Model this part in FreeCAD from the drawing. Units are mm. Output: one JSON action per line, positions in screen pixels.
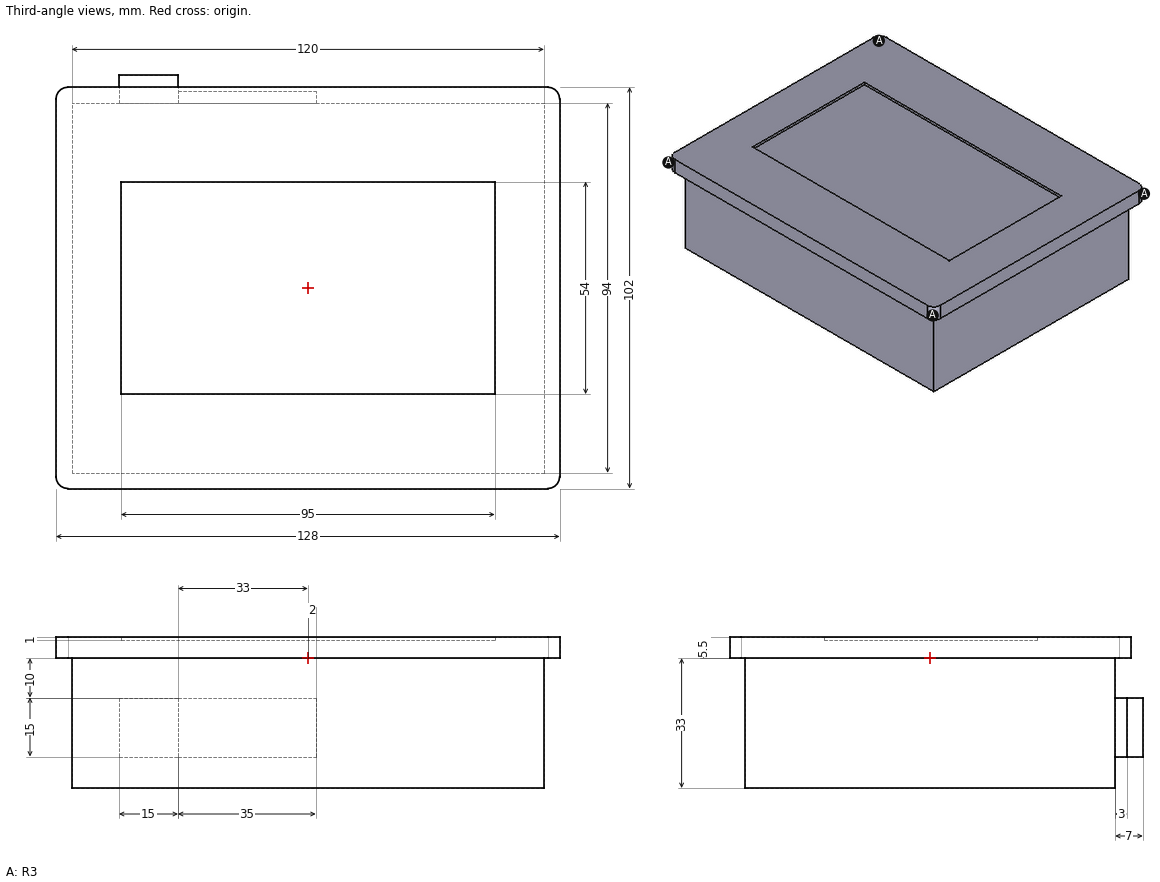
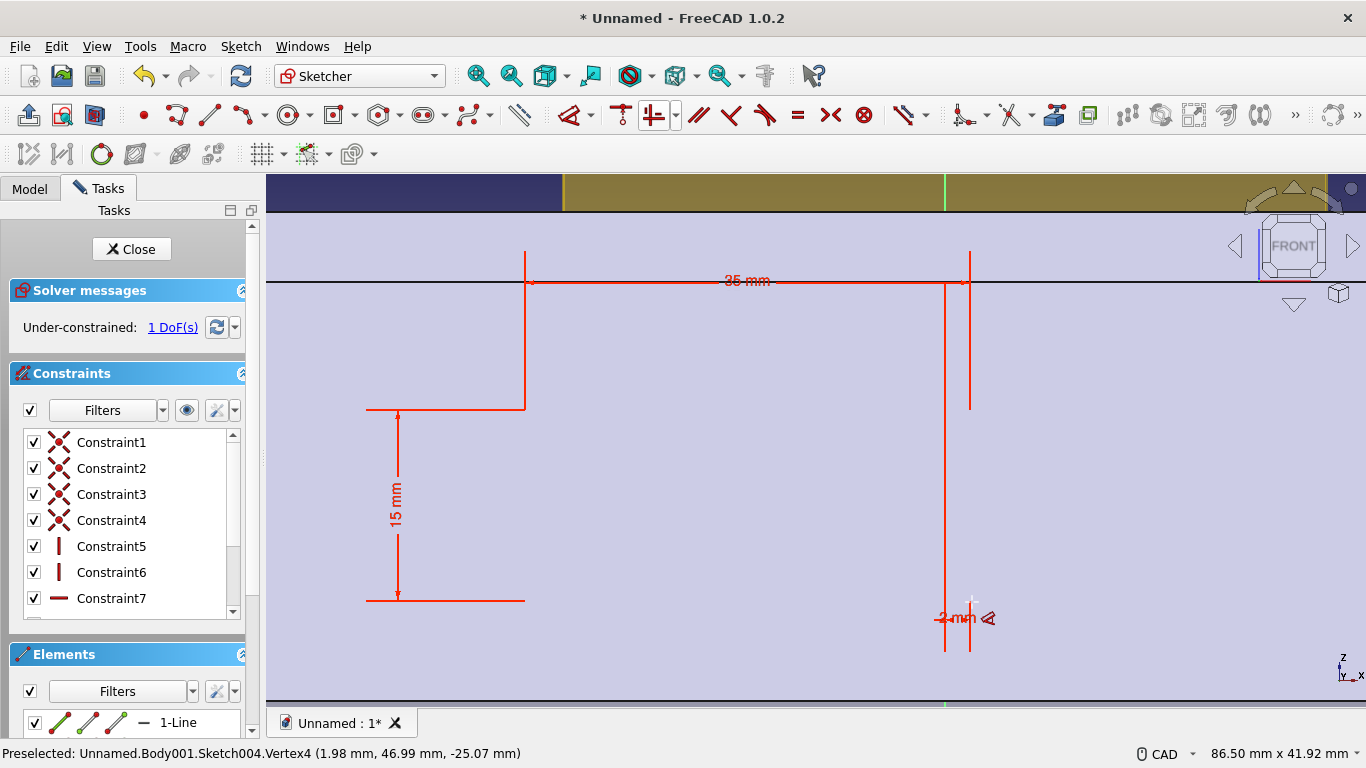
{"action": "left_click", "coordinate": [525, 410]}
{"action": "left_click", "coordinate": [491, 346]}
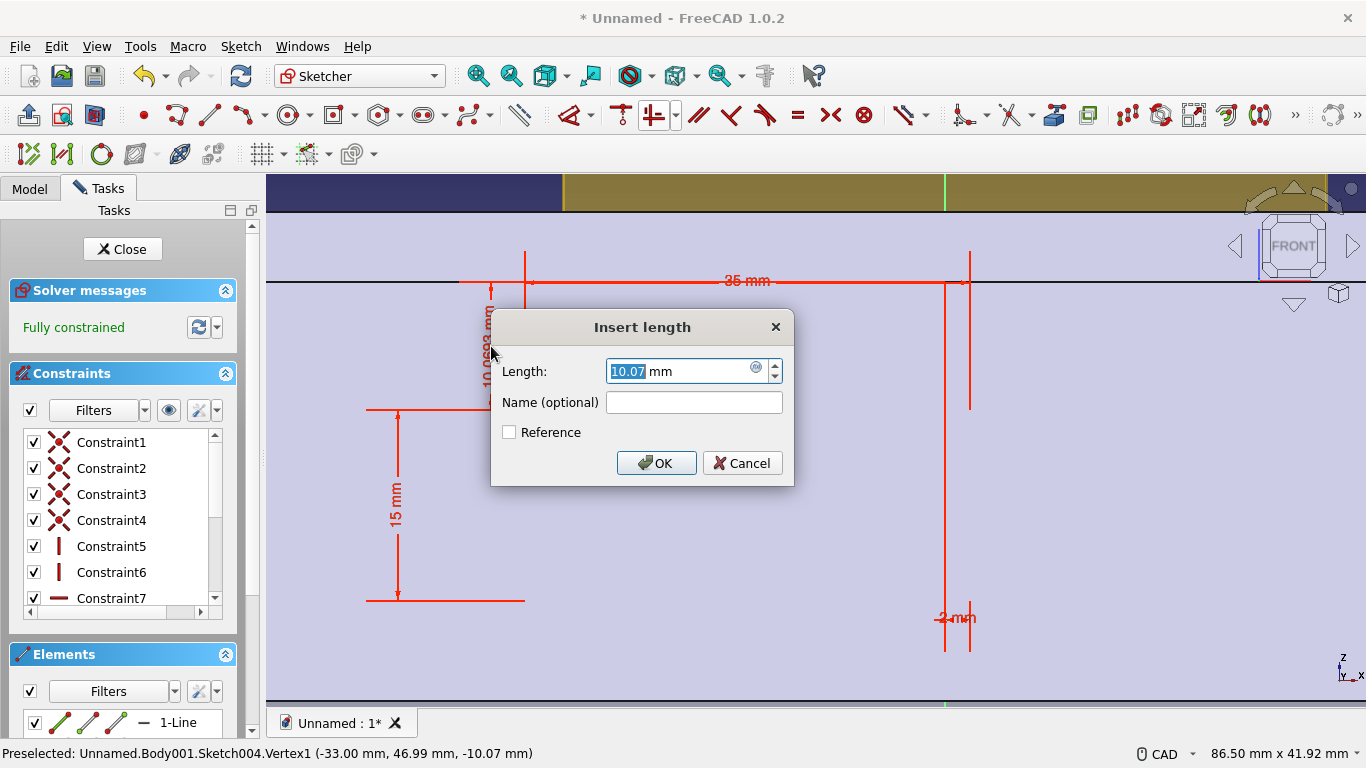
{"action": "type", "text": "10"}
{"action": "key", "text": "Return"}
{"action": "key", "text": "Escape"}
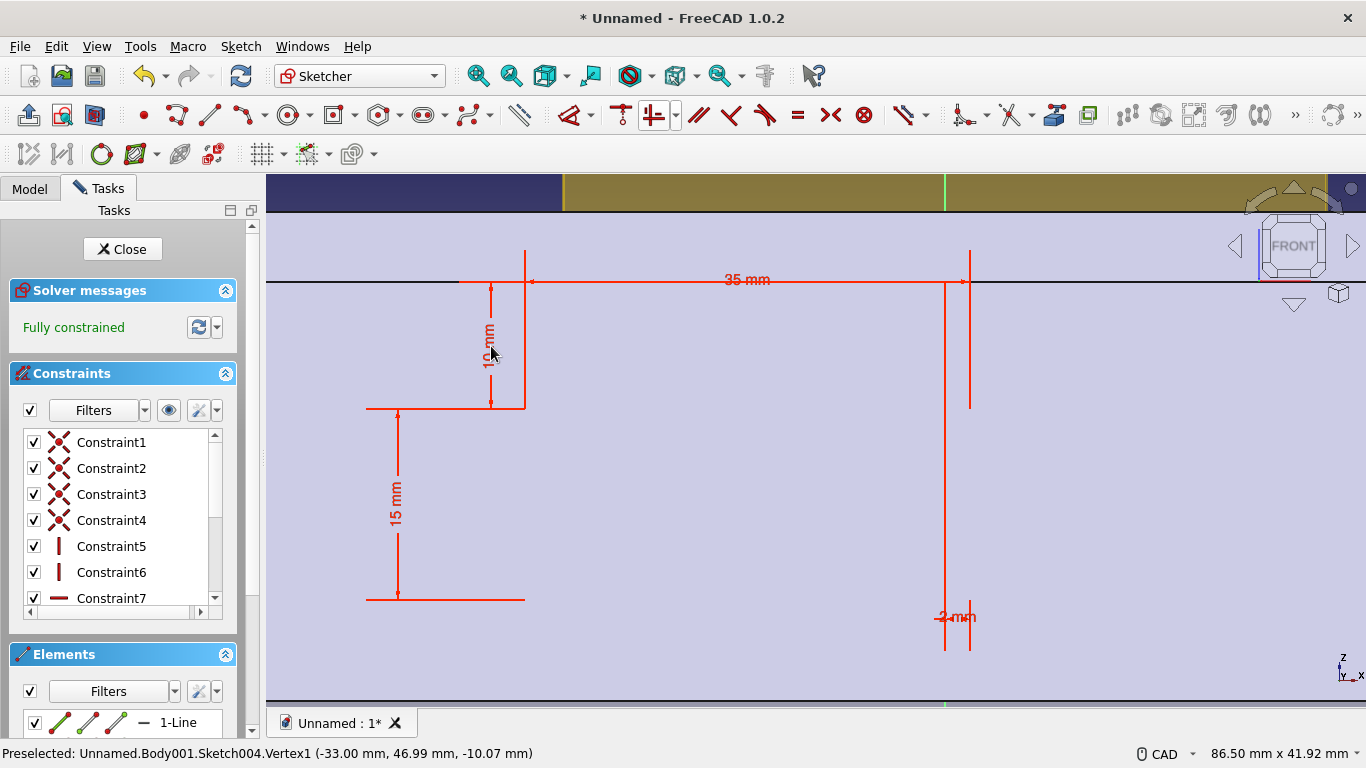
{"action": "left_click", "coordinate": [123, 249]}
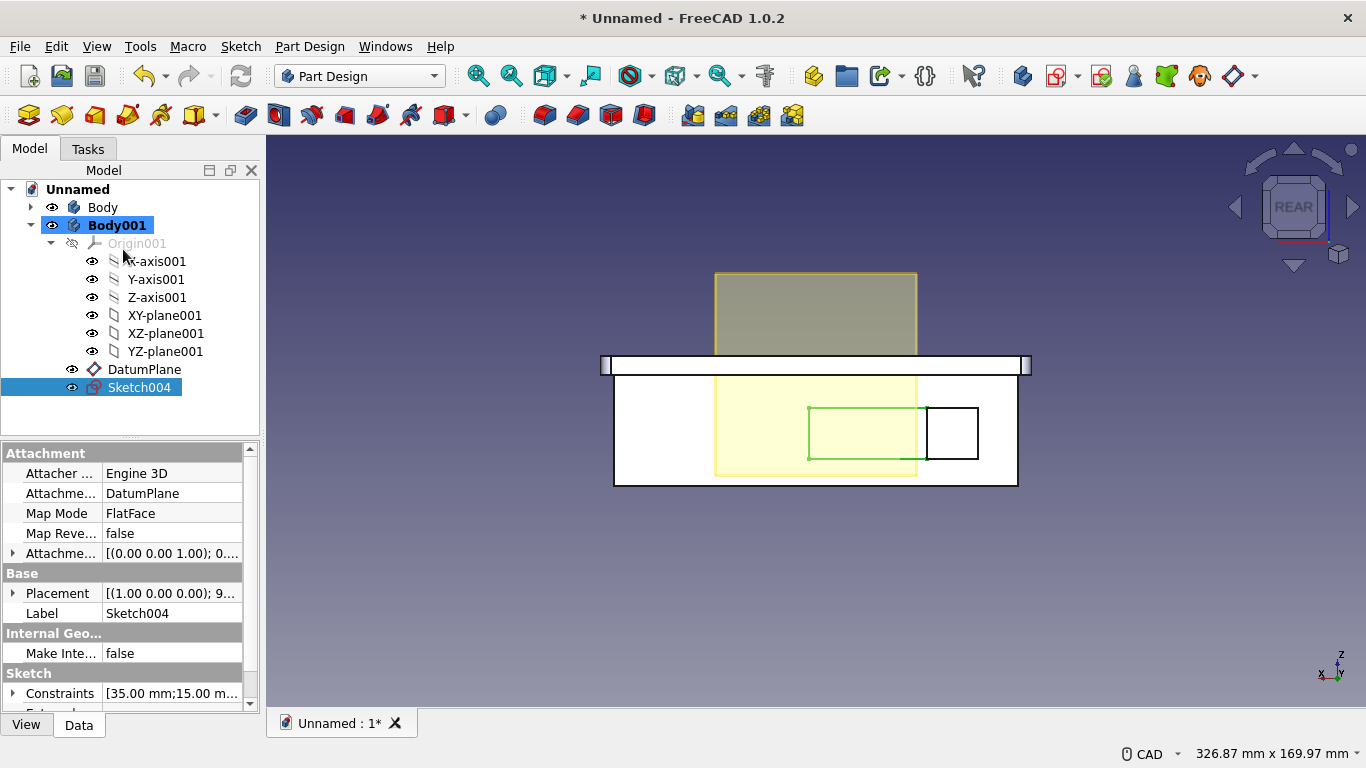
{"action": "left_click", "coordinate": [29, 116]}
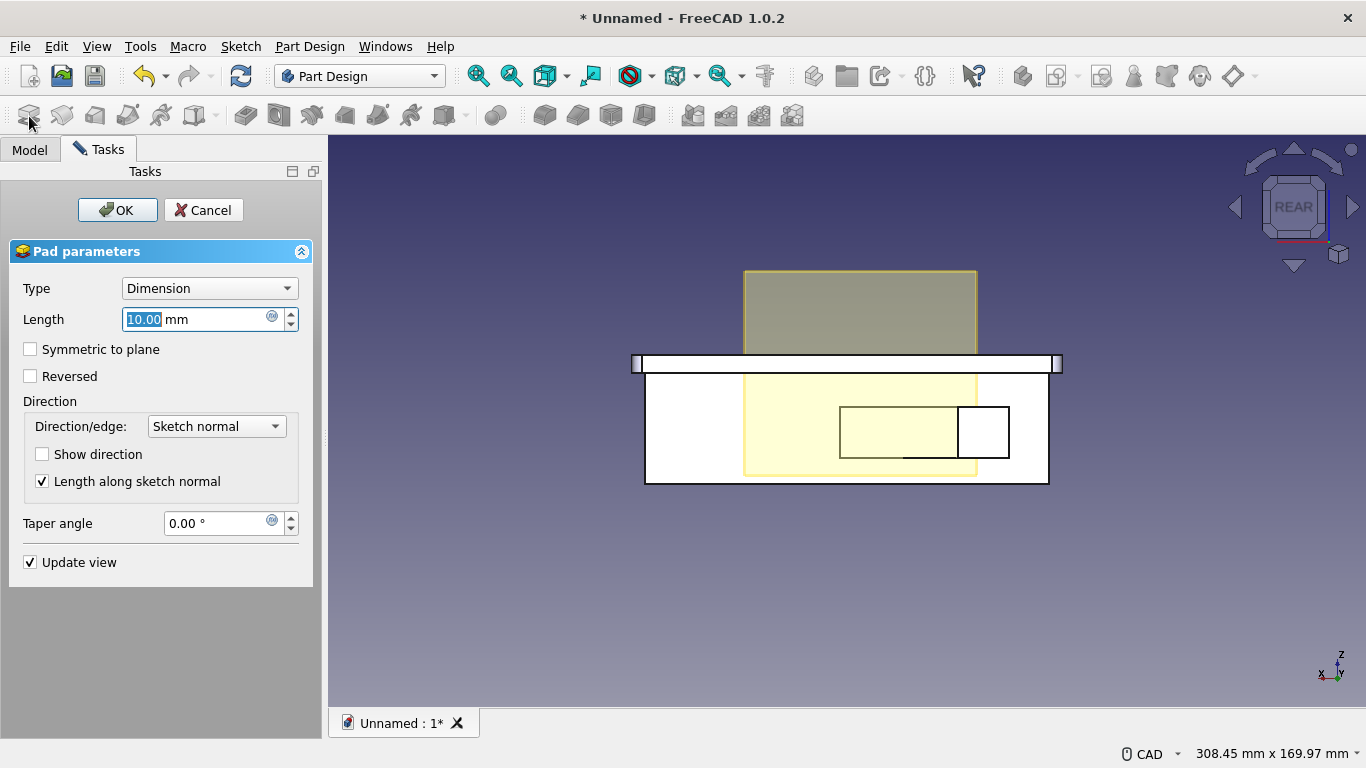
{"action": "type", "text": "3"}
{"action": "key", "text": "Tab"}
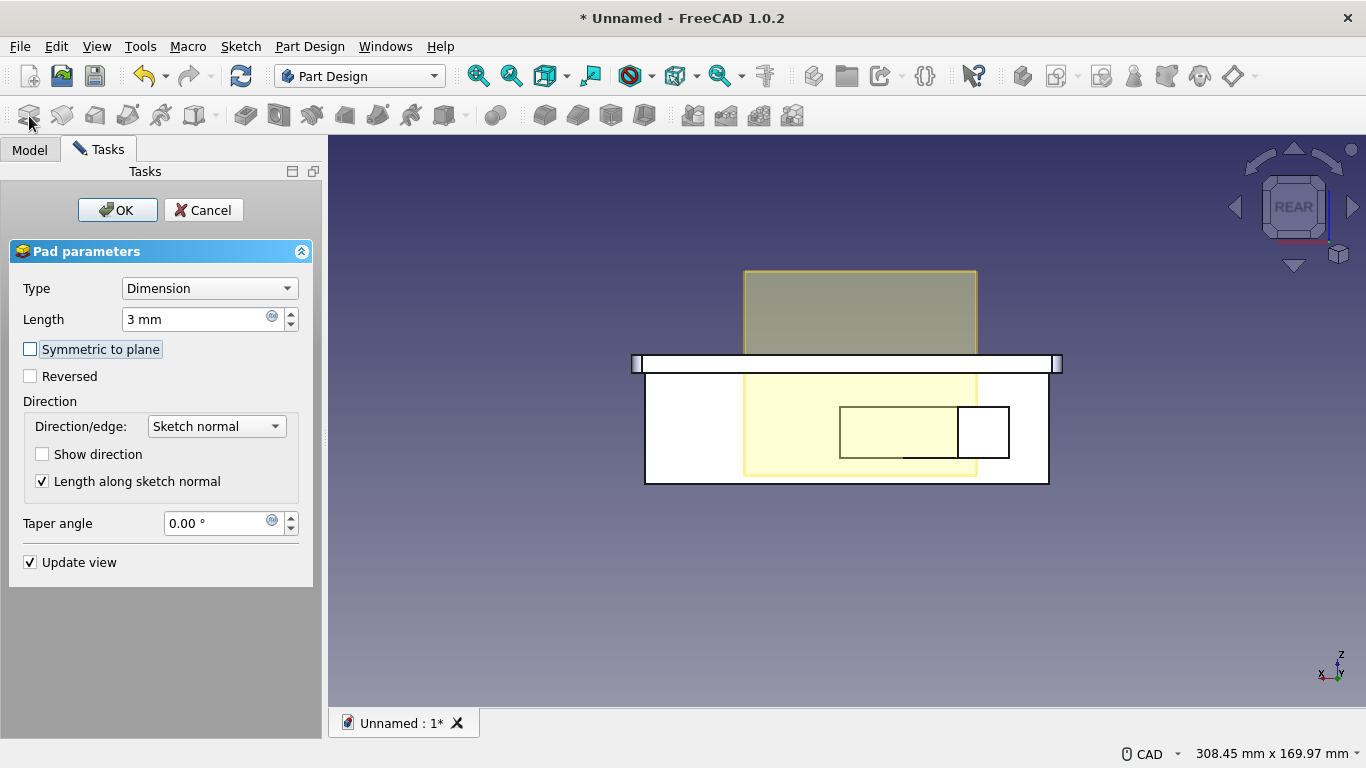
{"action": "left_click", "coordinate": [31, 376]}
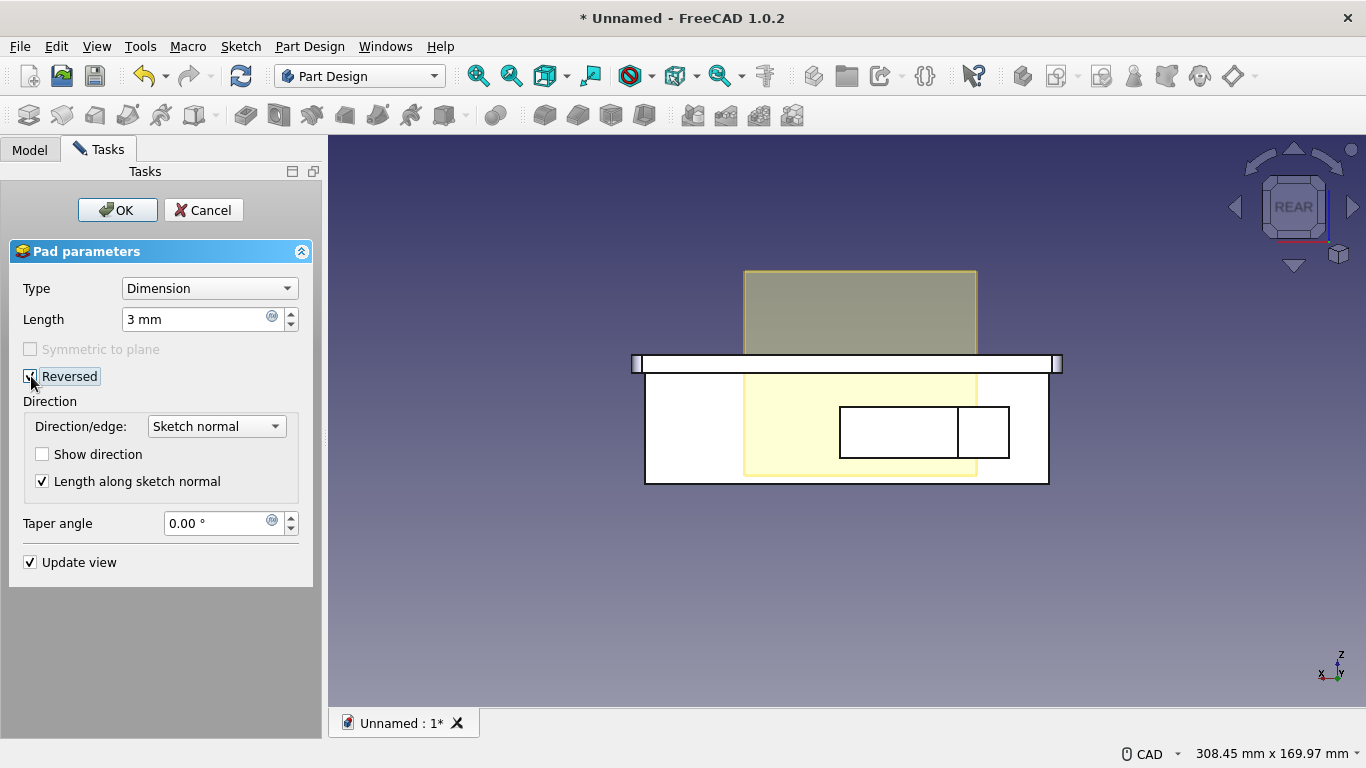
{"action": "left_click", "coordinate": [118, 210]}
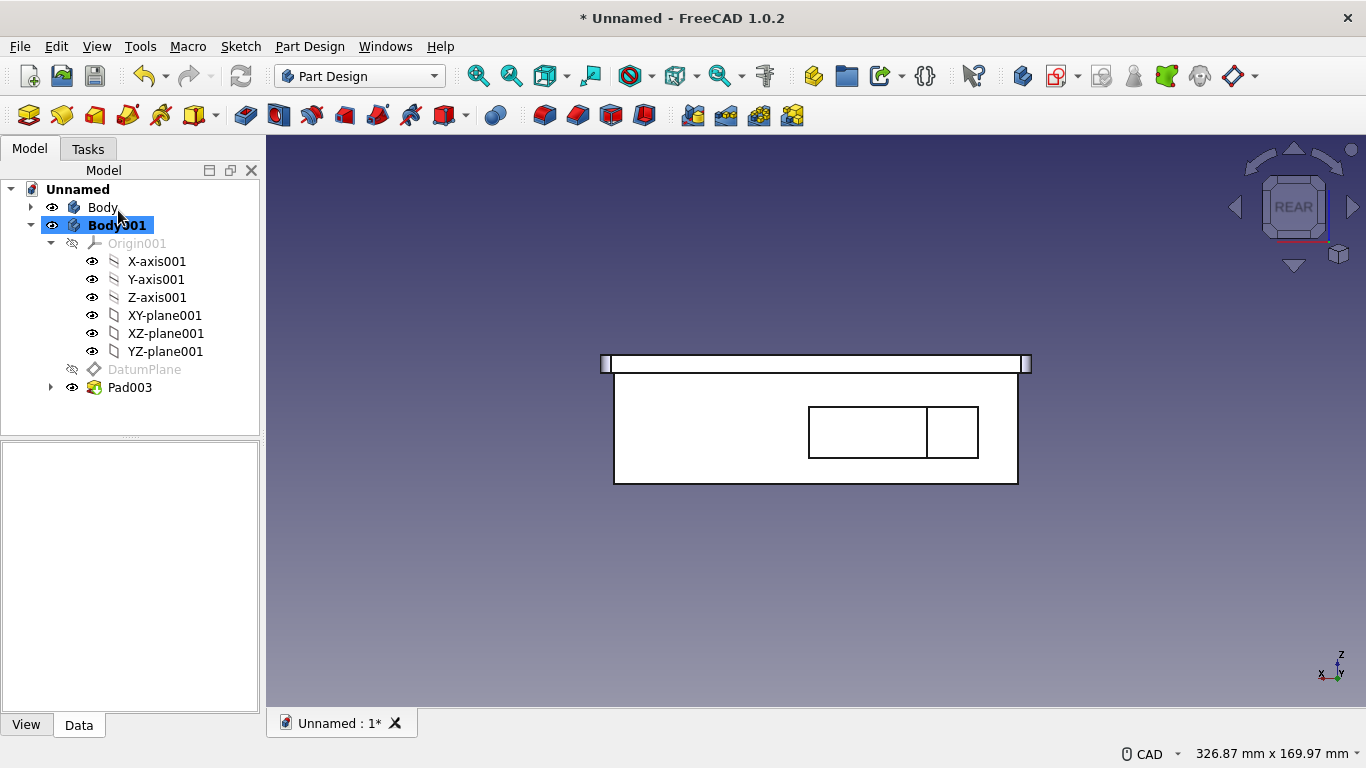
{"action": "key", "text": "0"}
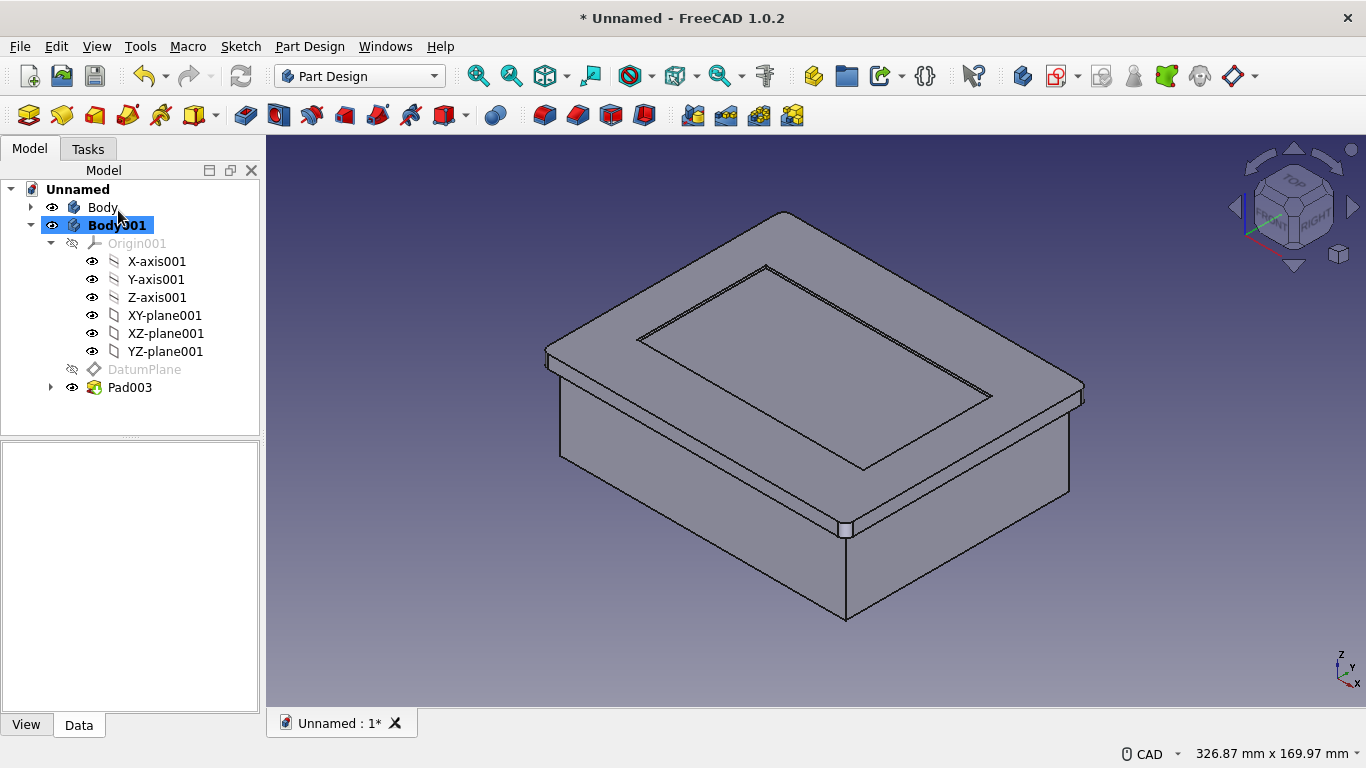
{"action": "left_click", "coordinate": [479, 76]}